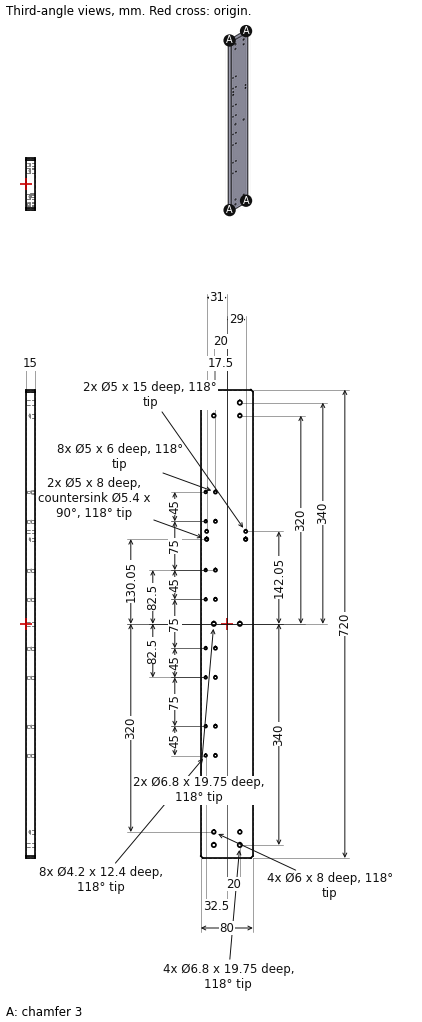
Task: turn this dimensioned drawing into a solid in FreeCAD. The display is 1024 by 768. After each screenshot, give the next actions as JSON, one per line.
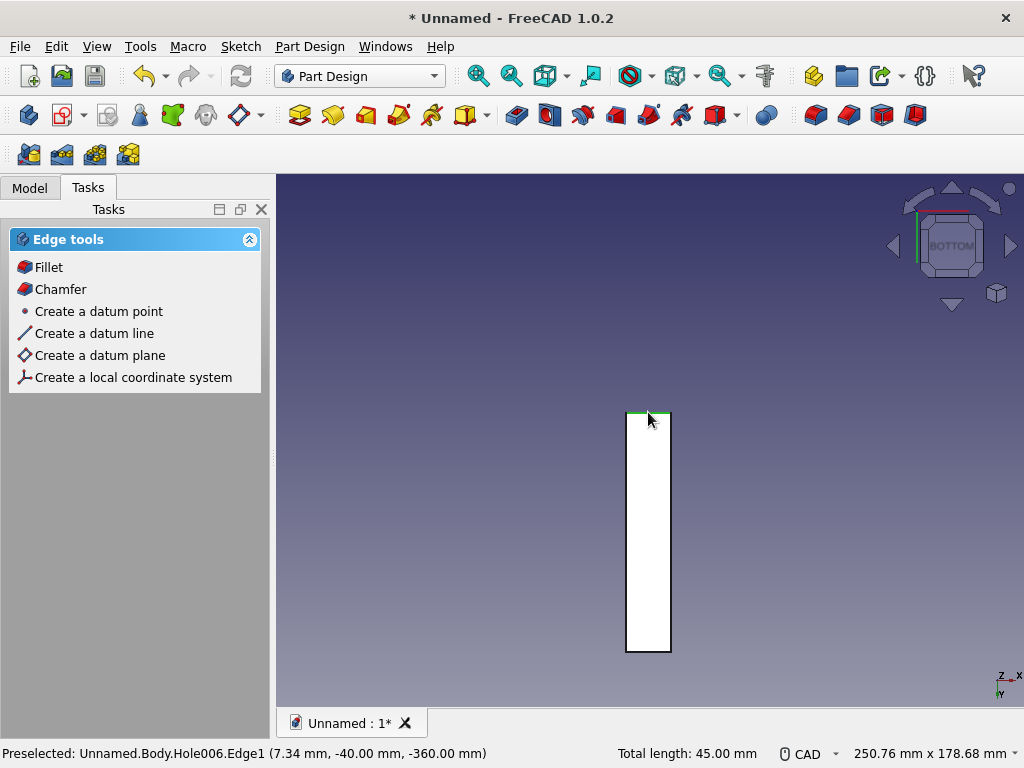
{"action": "left_click", "coordinate": [648, 651], "text": "ctrl"}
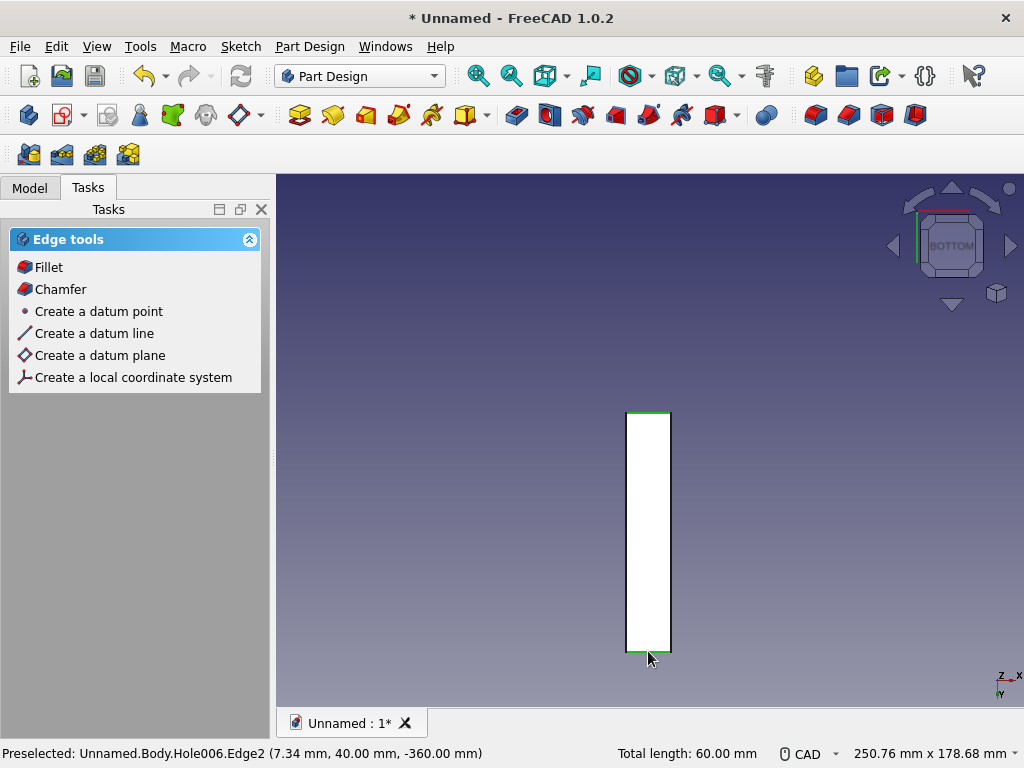
{"action": "left_click", "coordinate": [849, 116]}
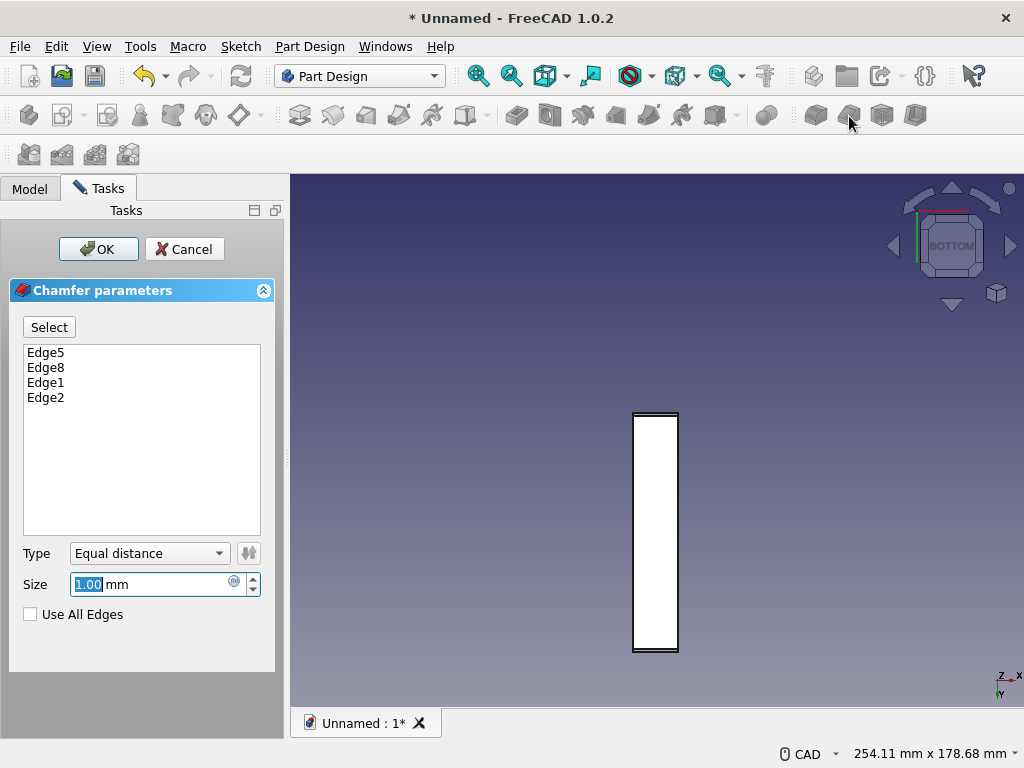
{"action": "type", "text": "3"}
{"action": "key", "text": "Tab"}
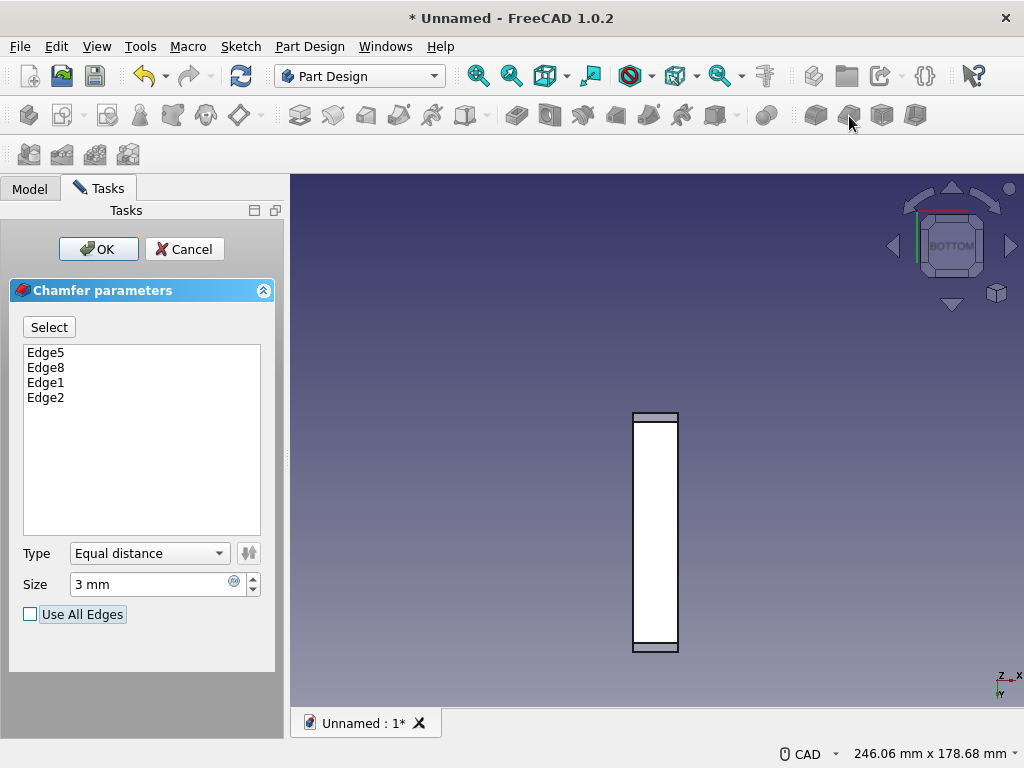
{"action": "left_click", "coordinate": [99, 249]}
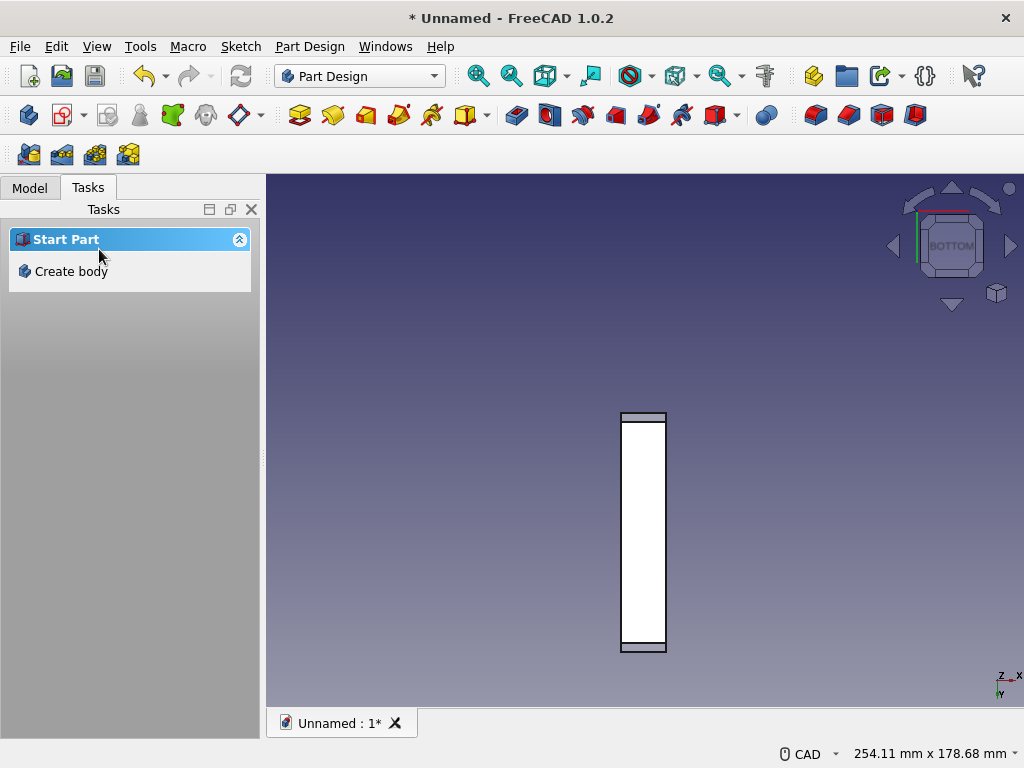
{"action": "key", "text": "0"}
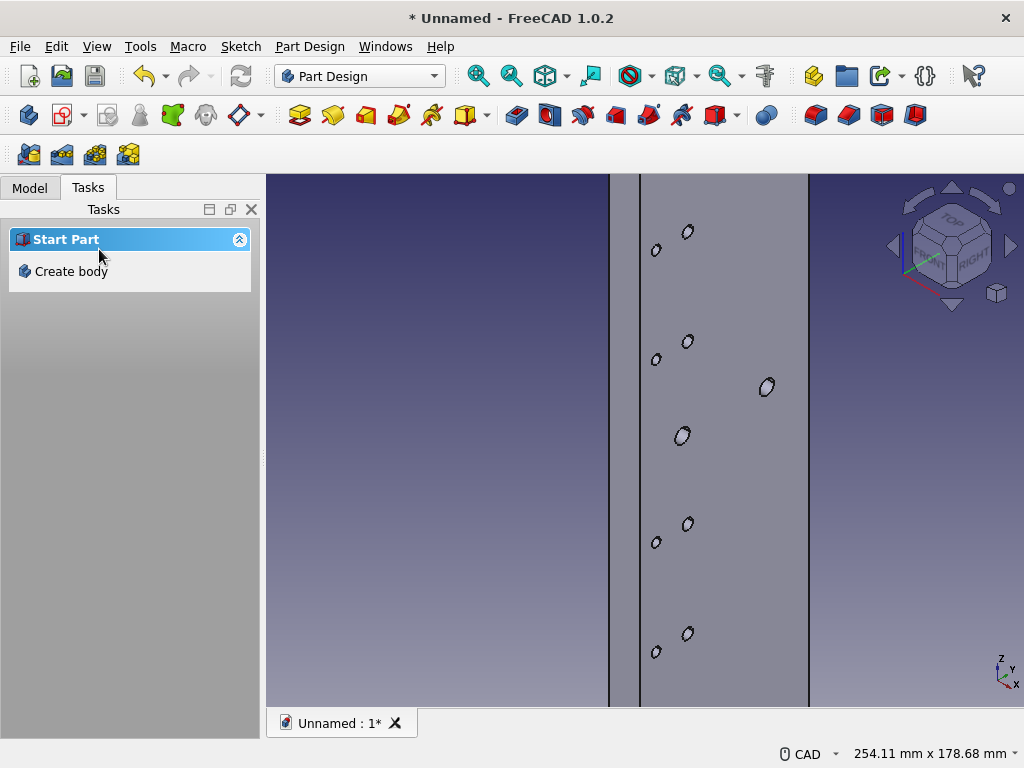
{"action": "left_click", "coordinate": [479, 76]}